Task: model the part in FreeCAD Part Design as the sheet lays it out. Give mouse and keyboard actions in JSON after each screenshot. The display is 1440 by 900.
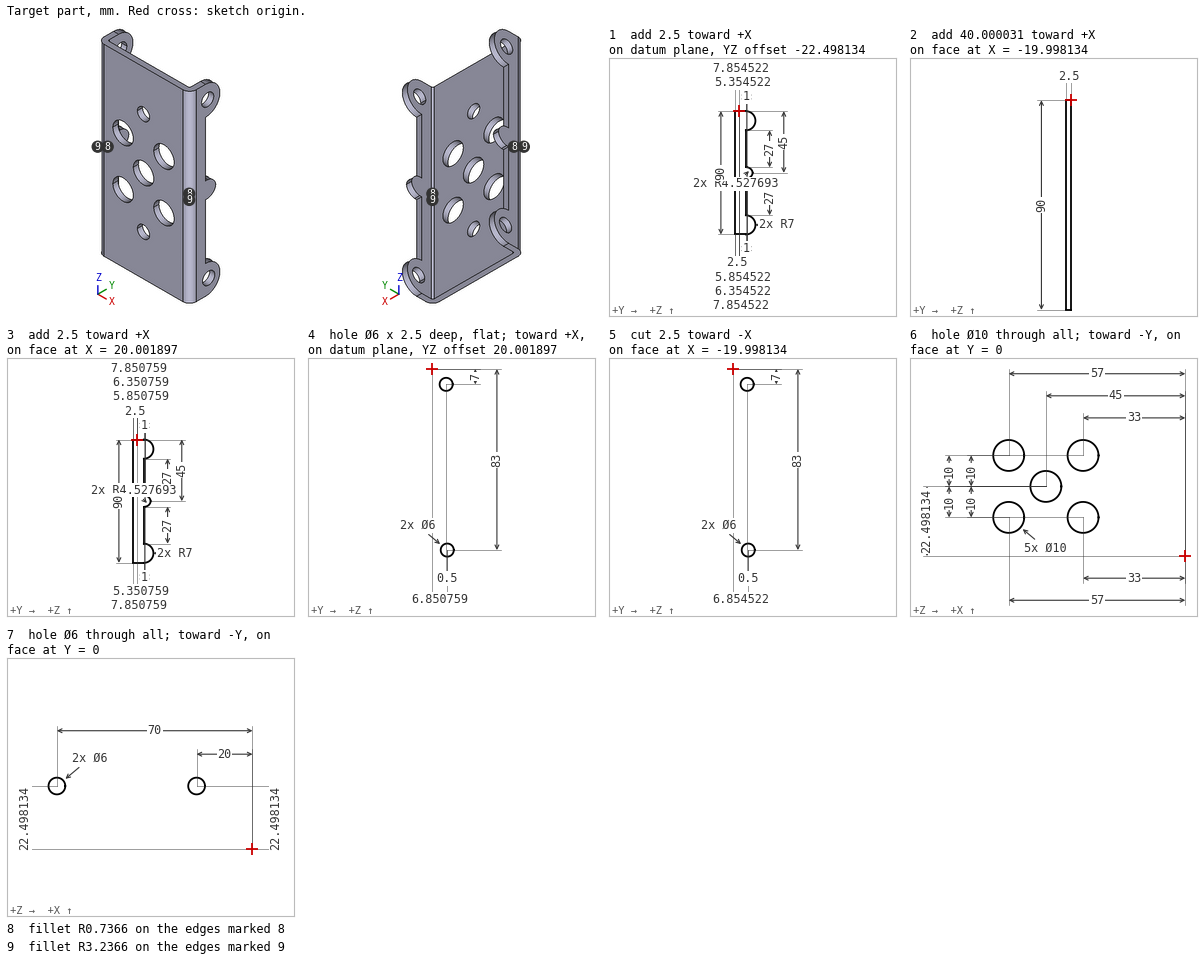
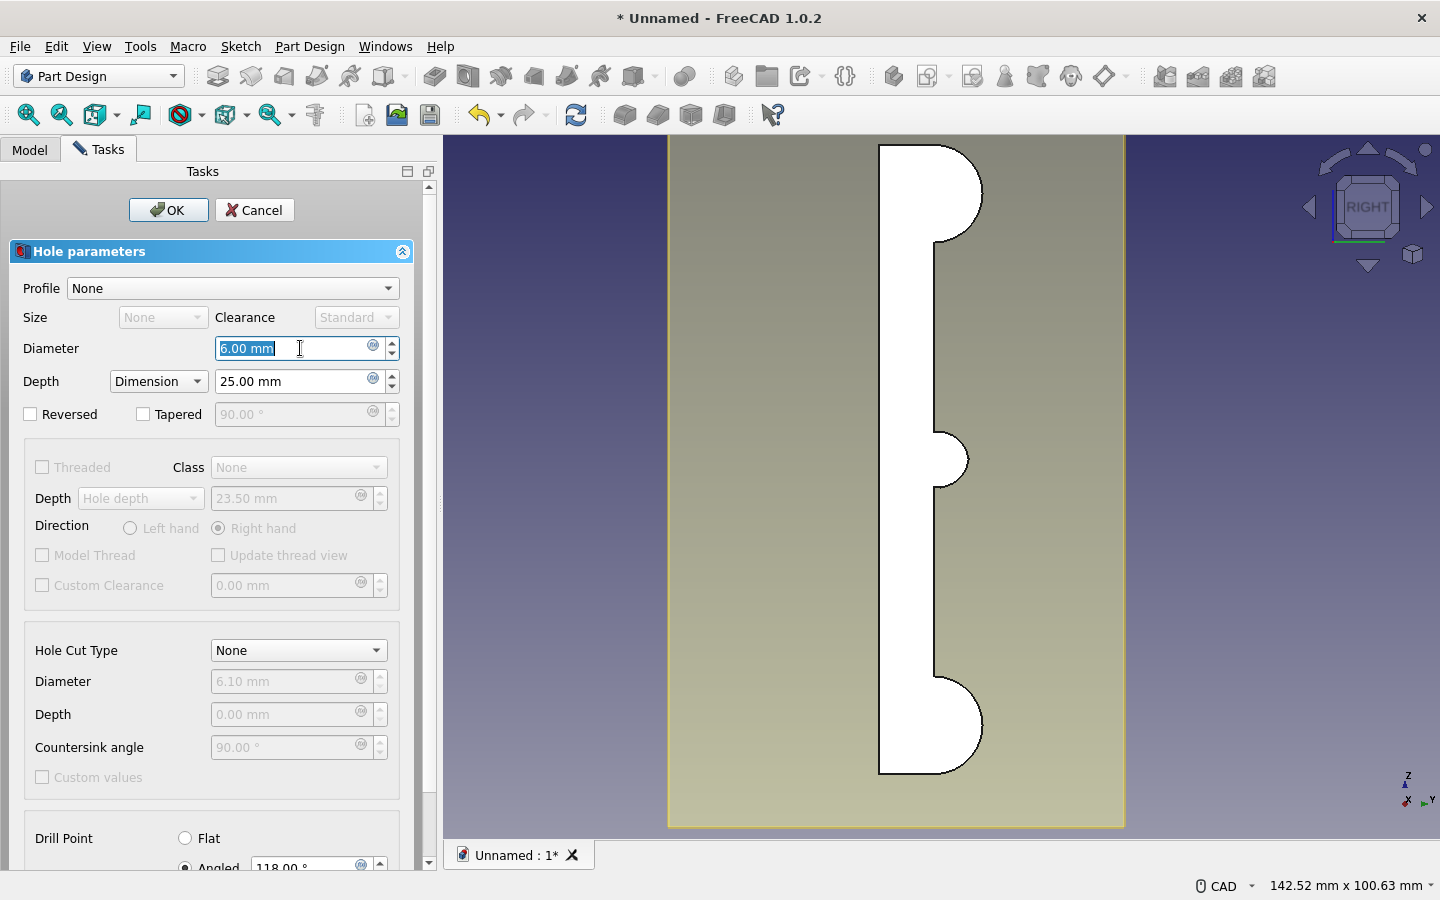
{"action": "type", "text": "6"}
{"action": "key", "text": "Tab"}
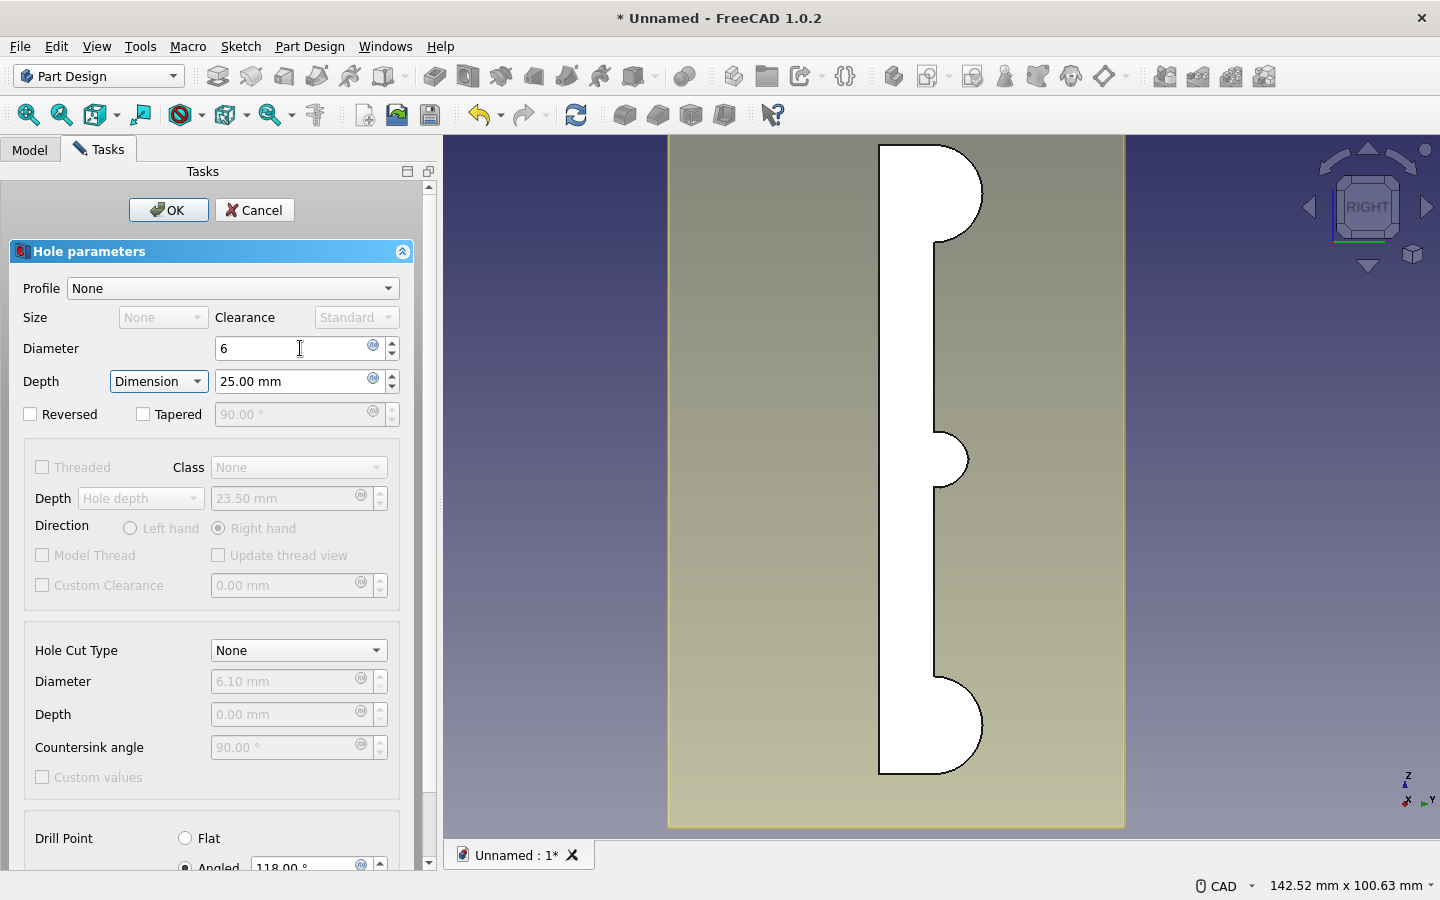
{"action": "triple_click", "coordinate": [300, 382]}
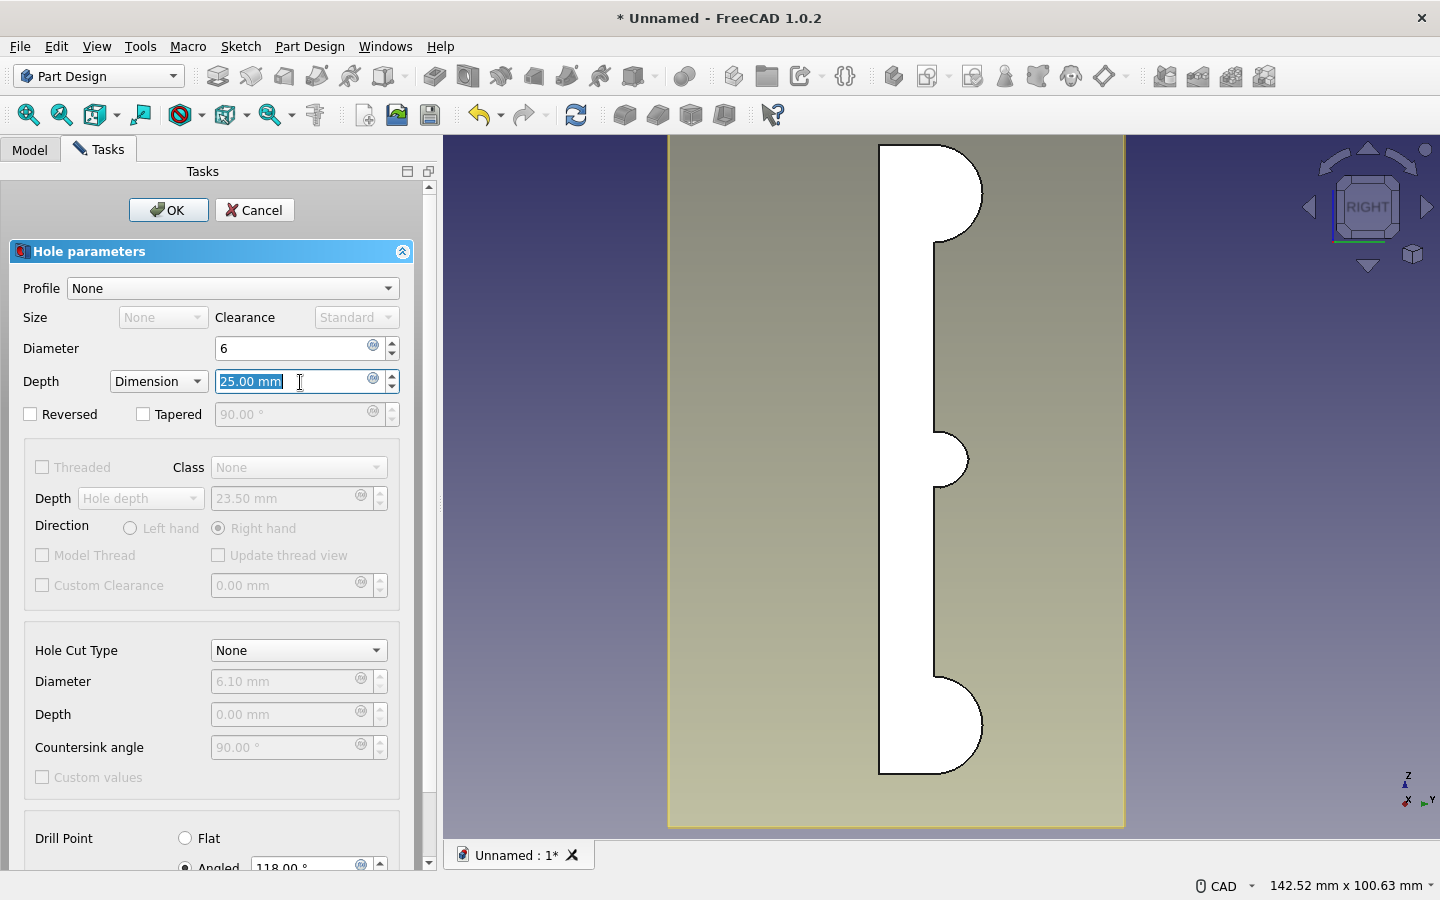
{"action": "type", "text": "2.5"}
{"action": "key", "text": "Tab"}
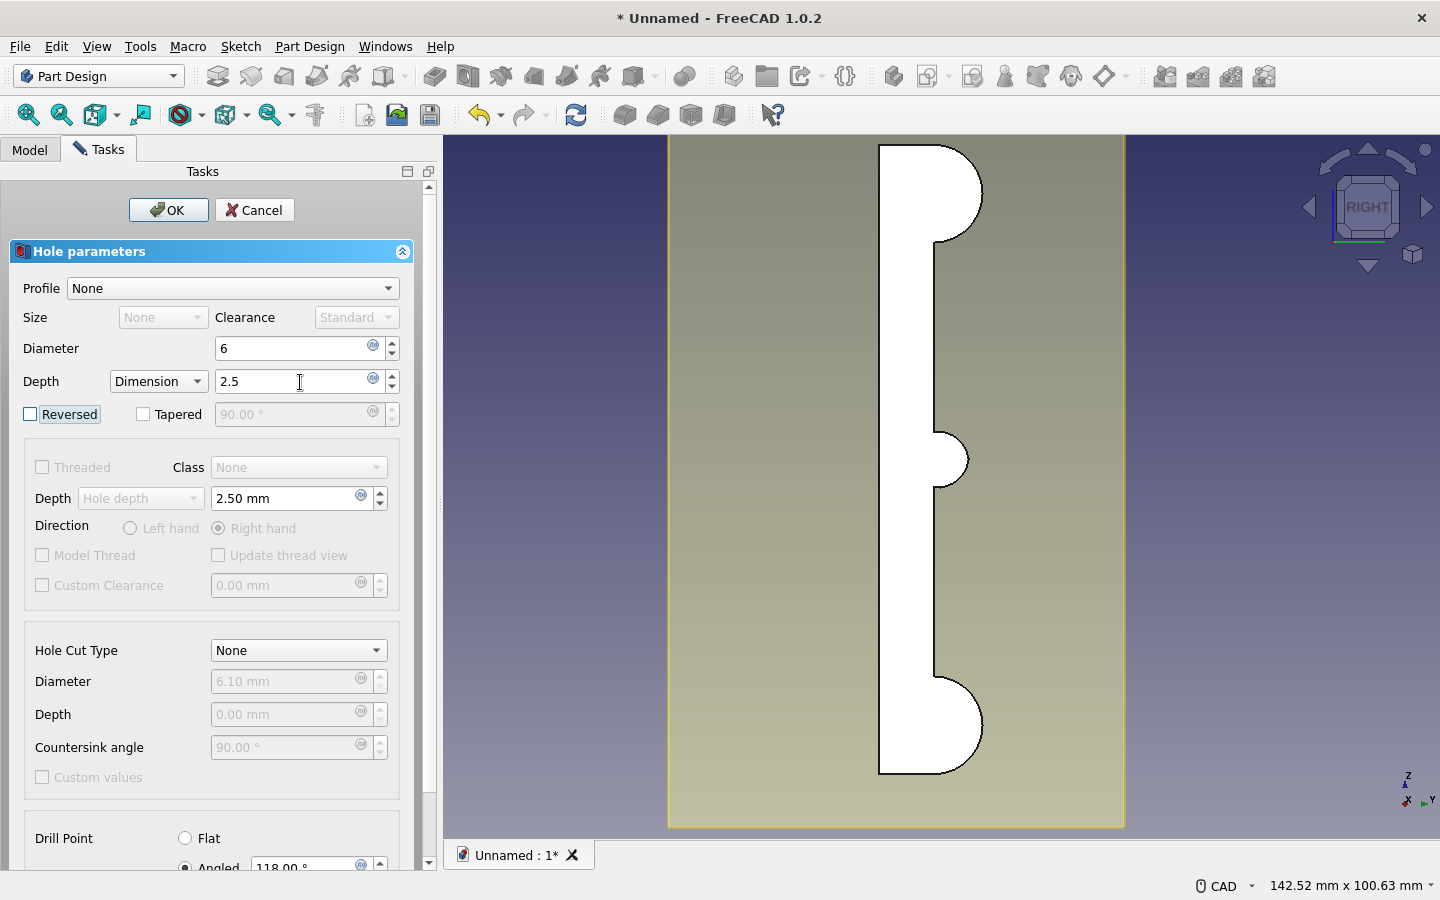
{"action": "left_click", "coordinate": [31, 414]}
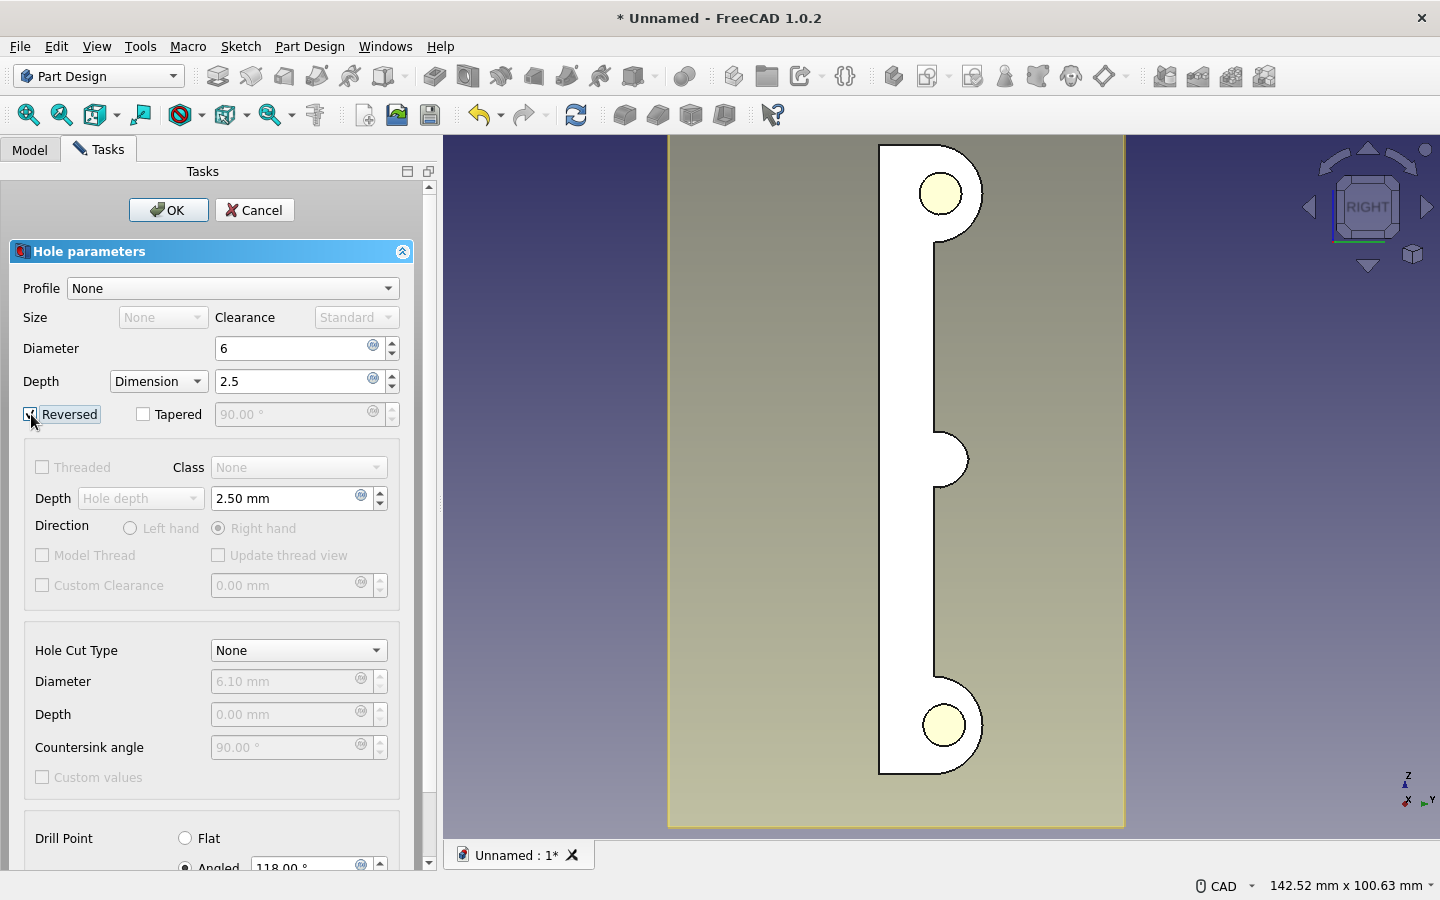
{"action": "left_click", "coordinate": [186, 836]}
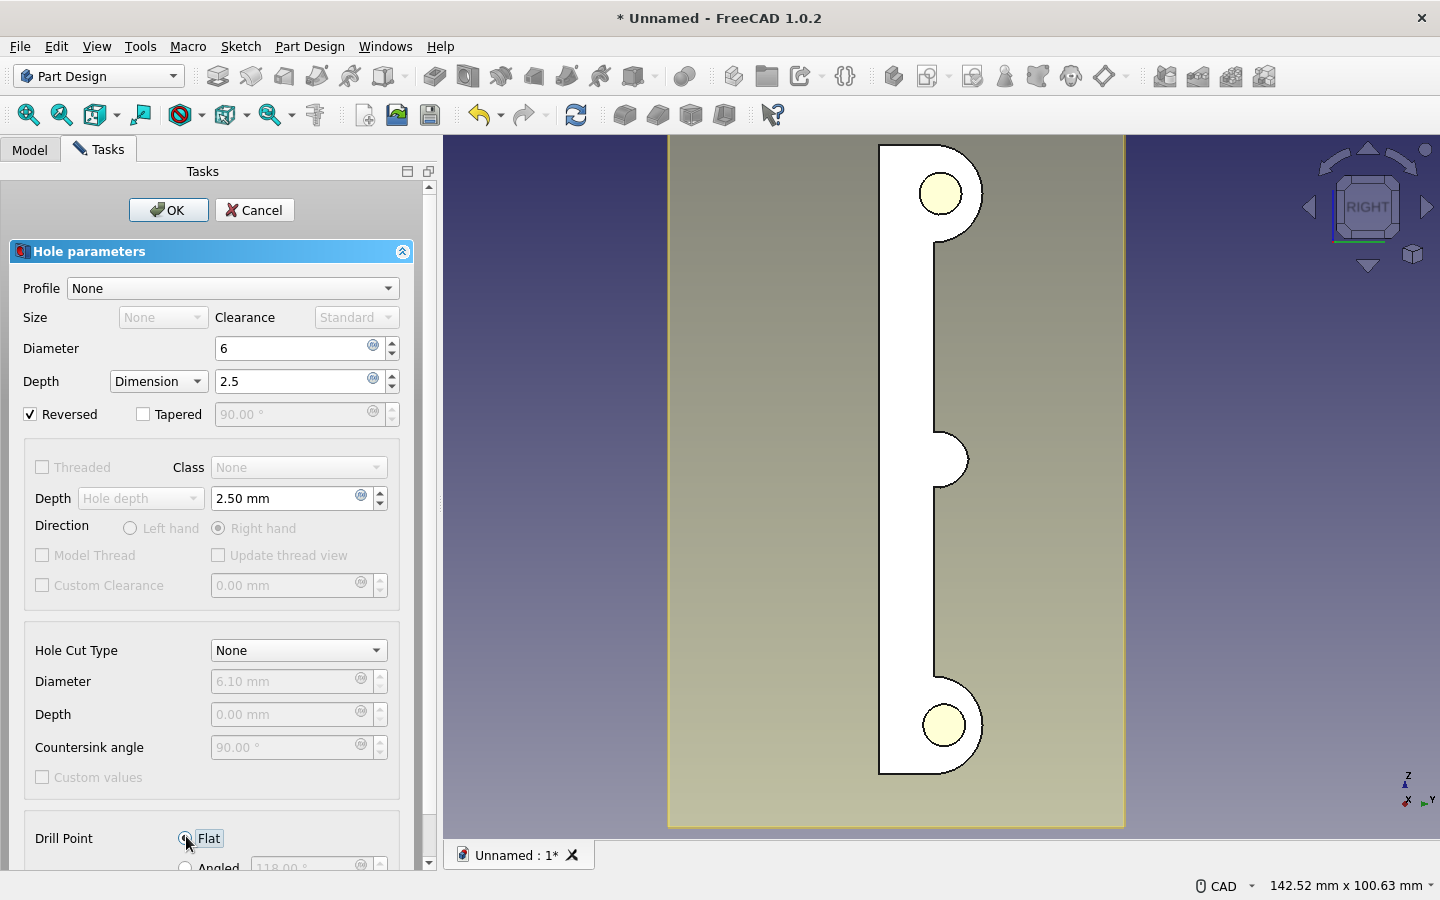
{"action": "left_click", "coordinate": [169, 210]}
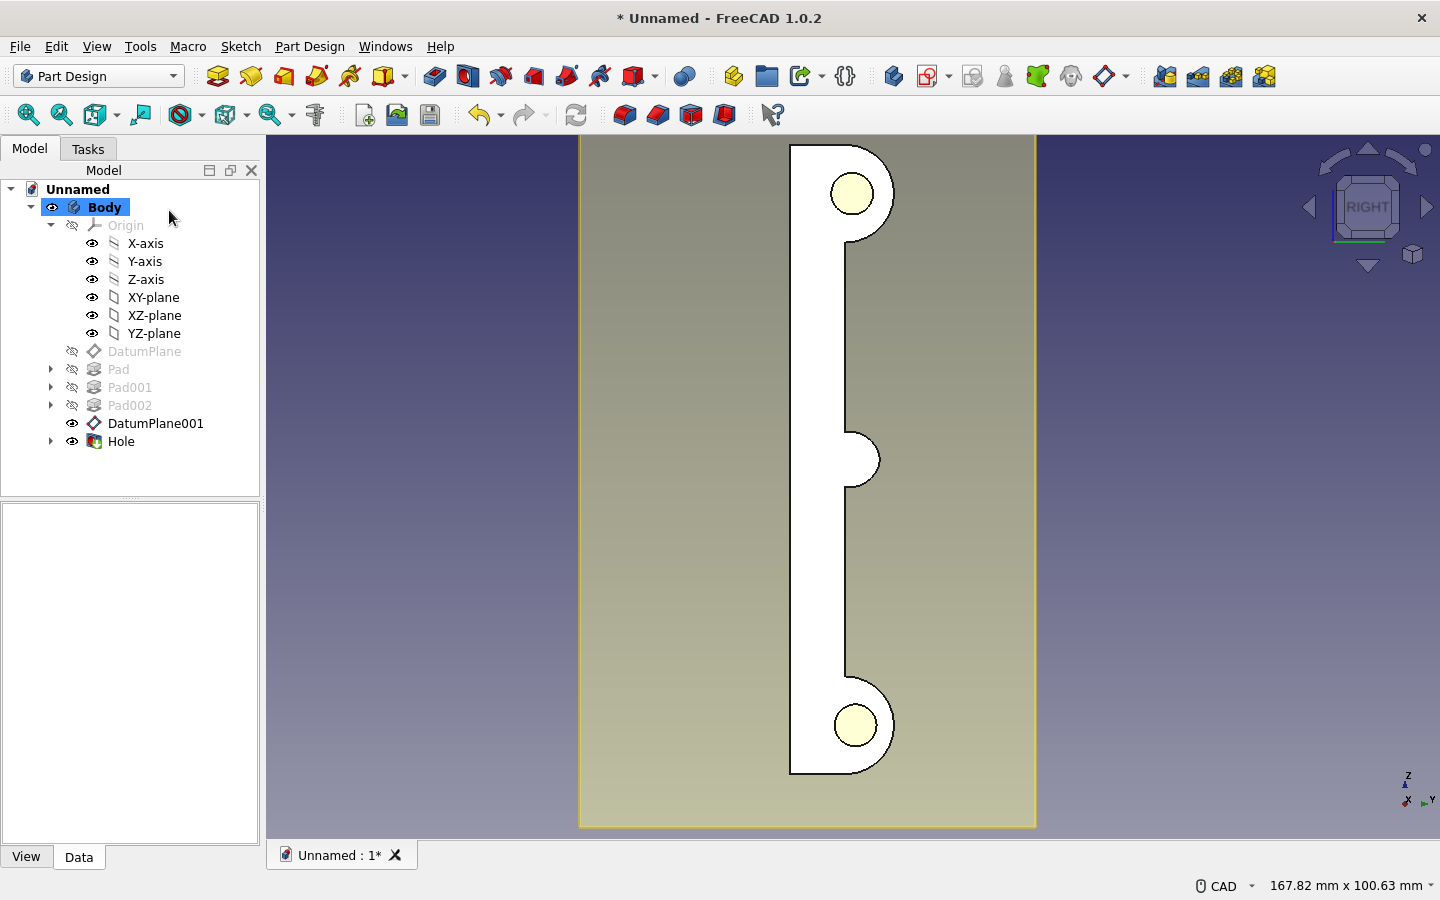
{"action": "left_click", "coordinate": [117, 423]}
{"action": "key", "text": "space"}